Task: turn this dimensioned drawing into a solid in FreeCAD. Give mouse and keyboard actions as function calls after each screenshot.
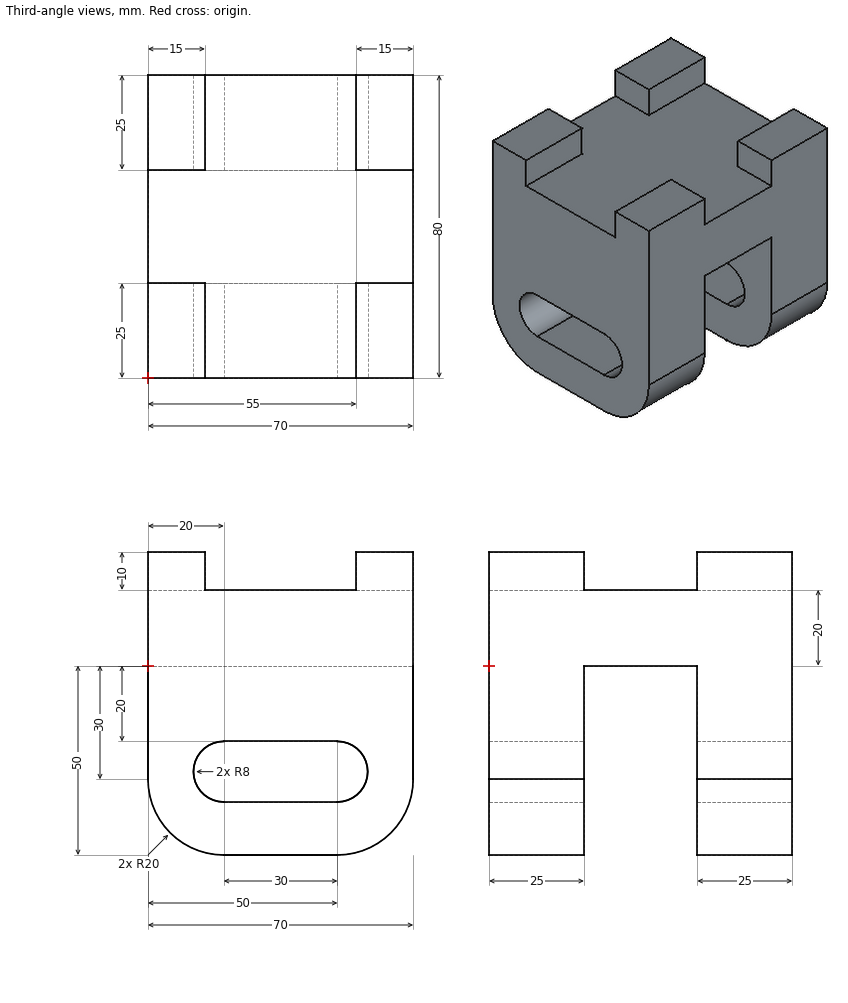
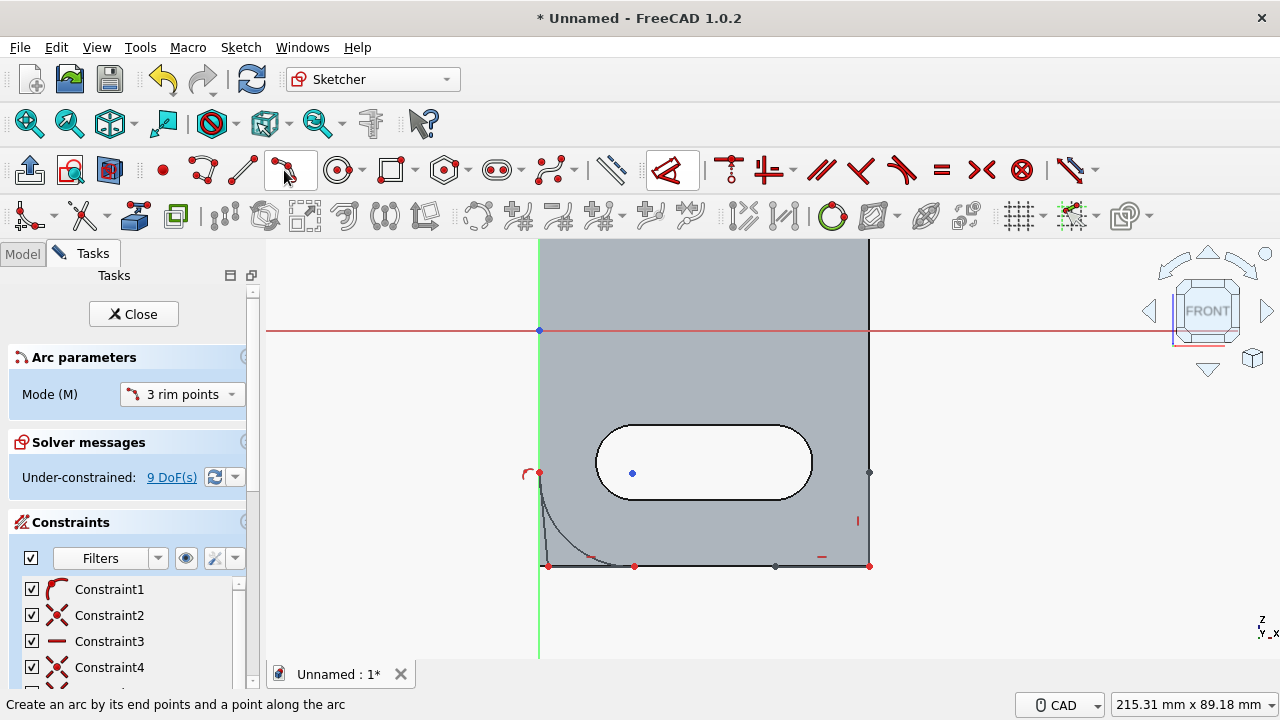
click(869, 473)
click(775, 567)
click(842, 539)
key(Escape)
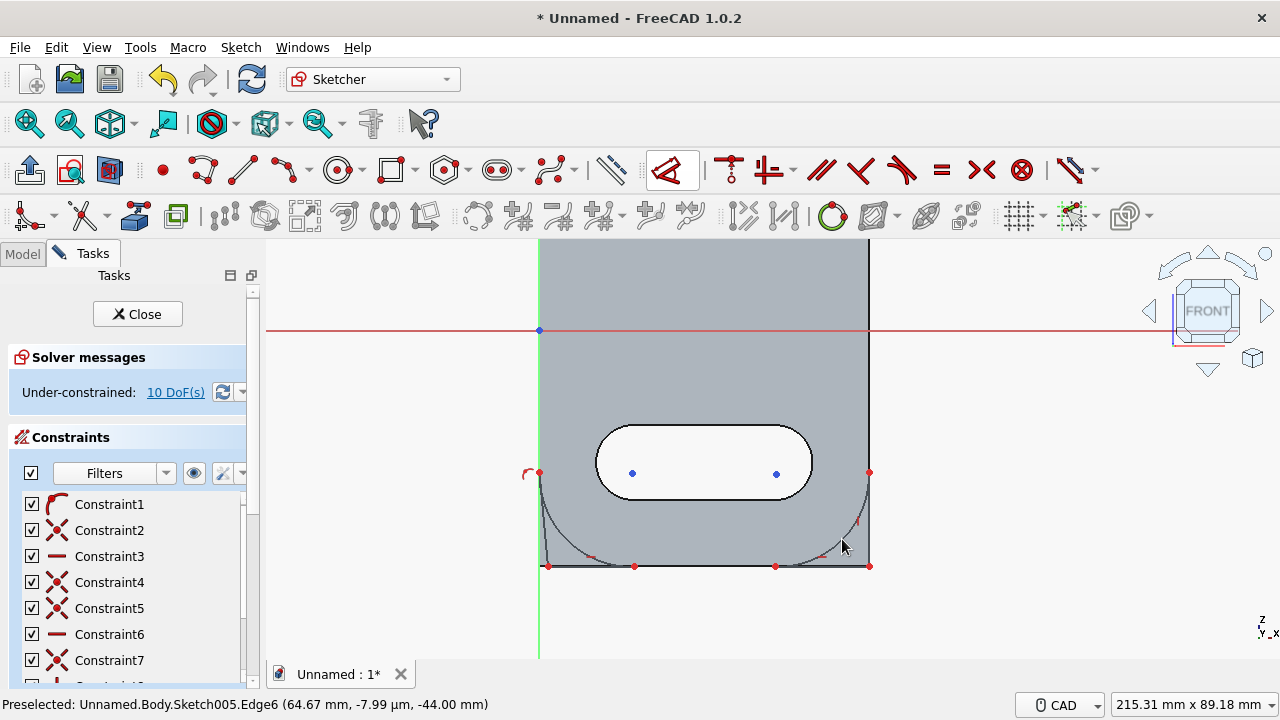
scroll(546, 548, up, 4)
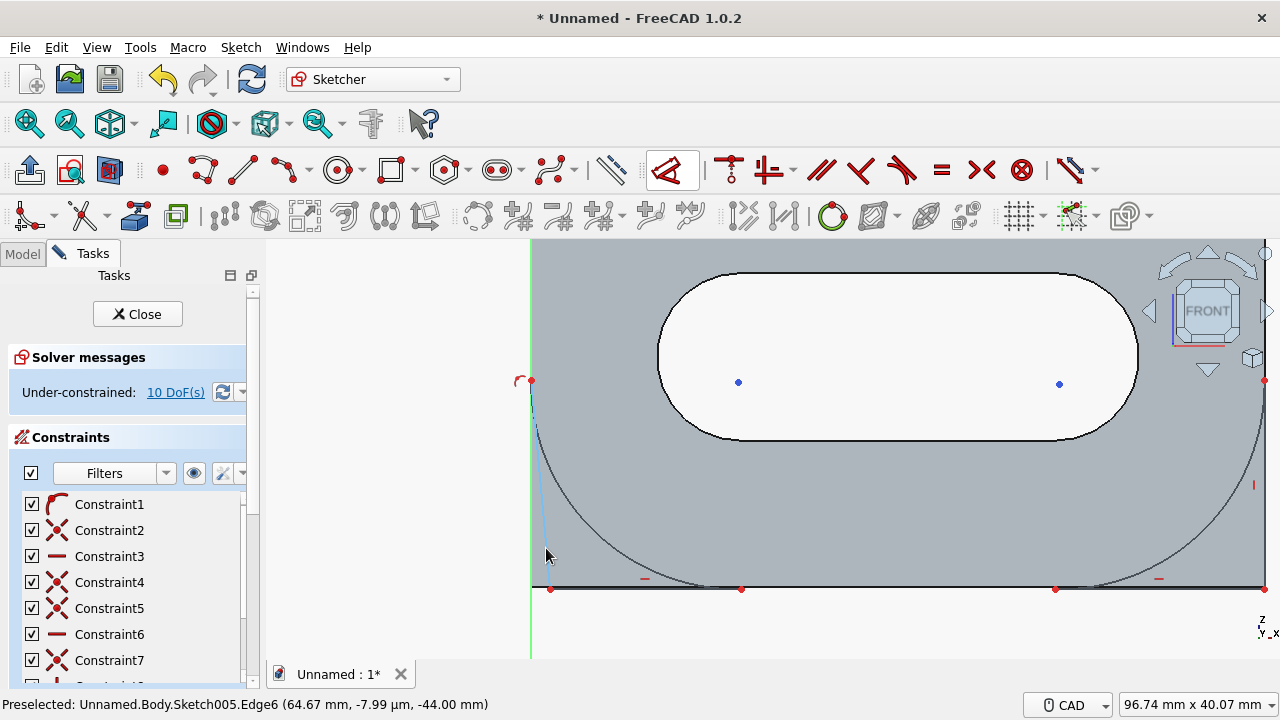
click(546, 548)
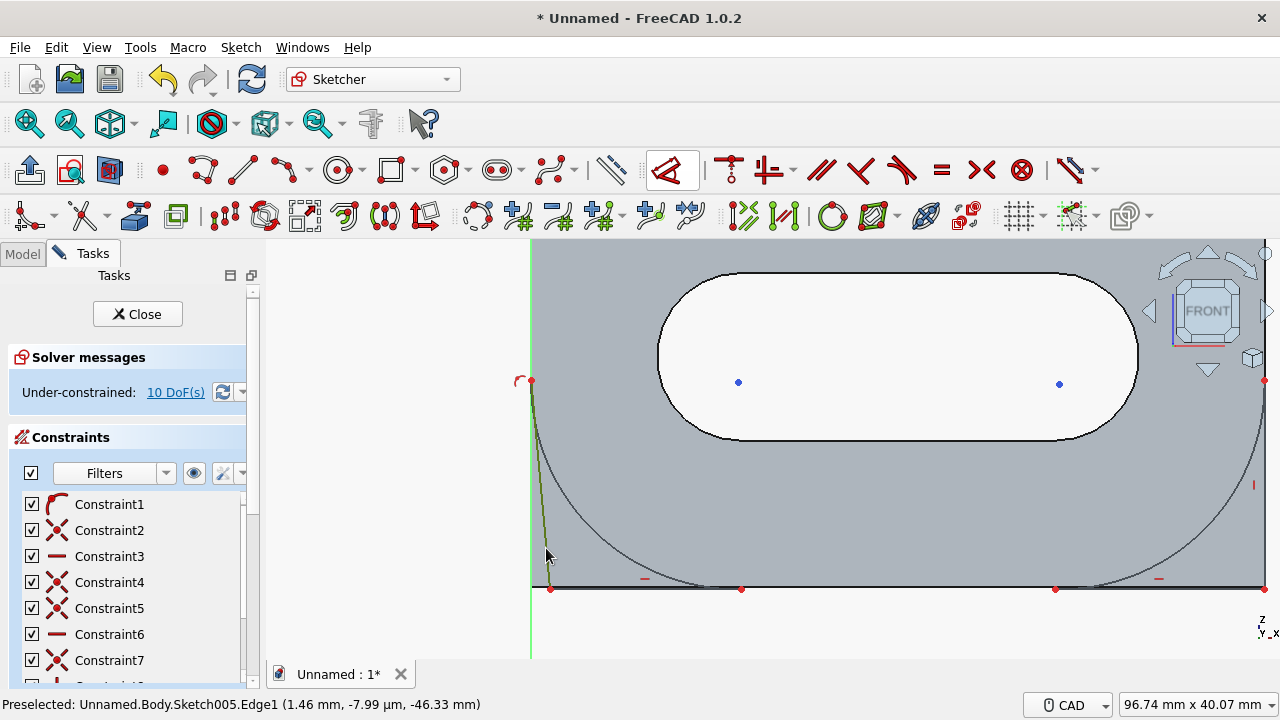
click(554, 476)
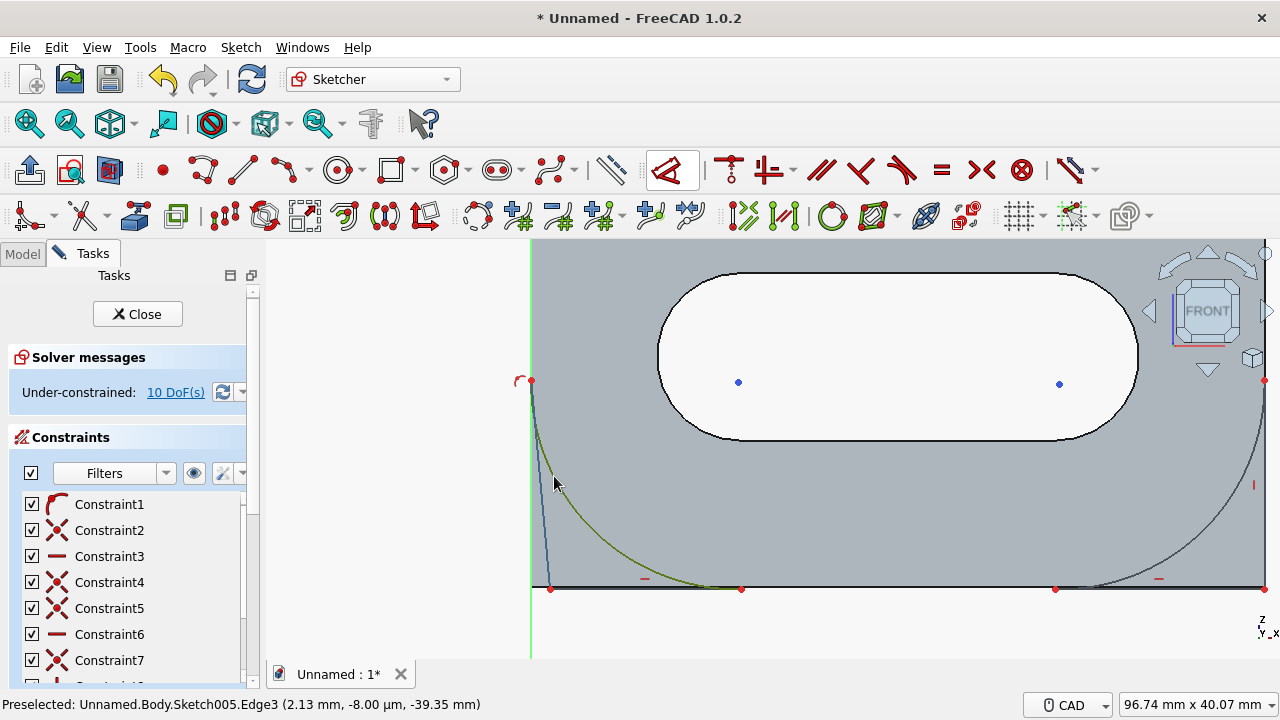
click(902, 170)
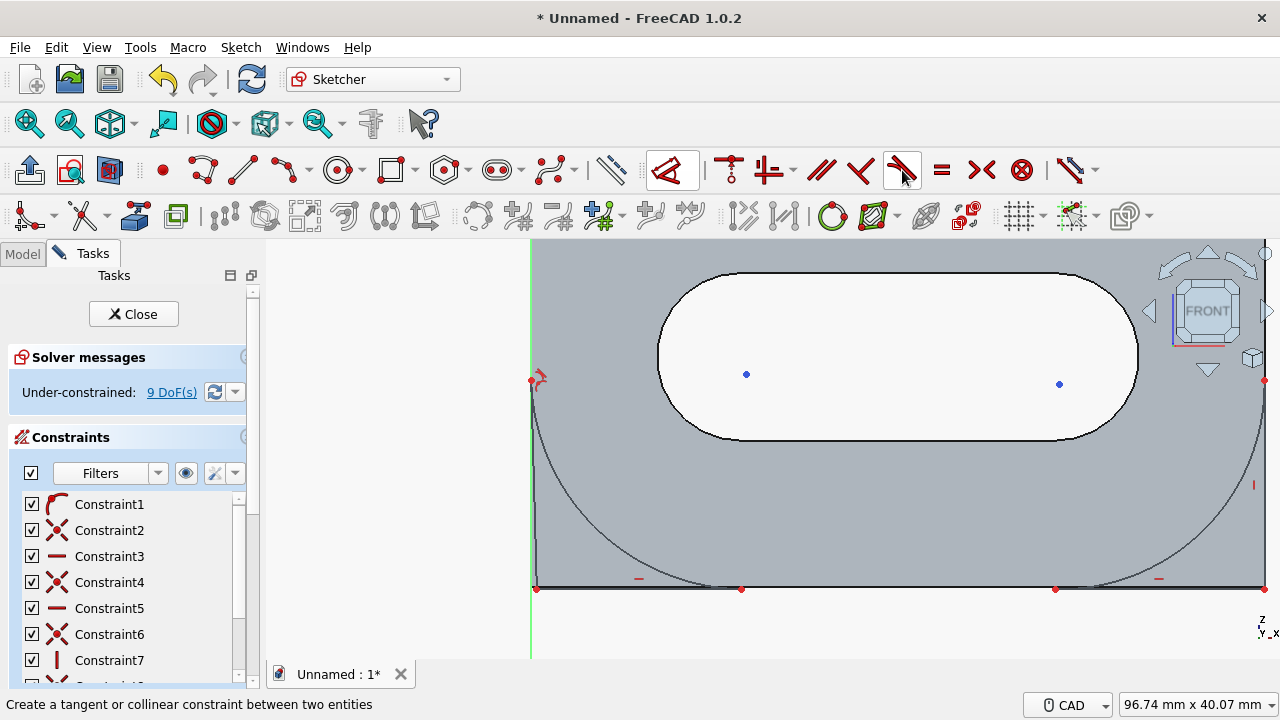
click(598, 589)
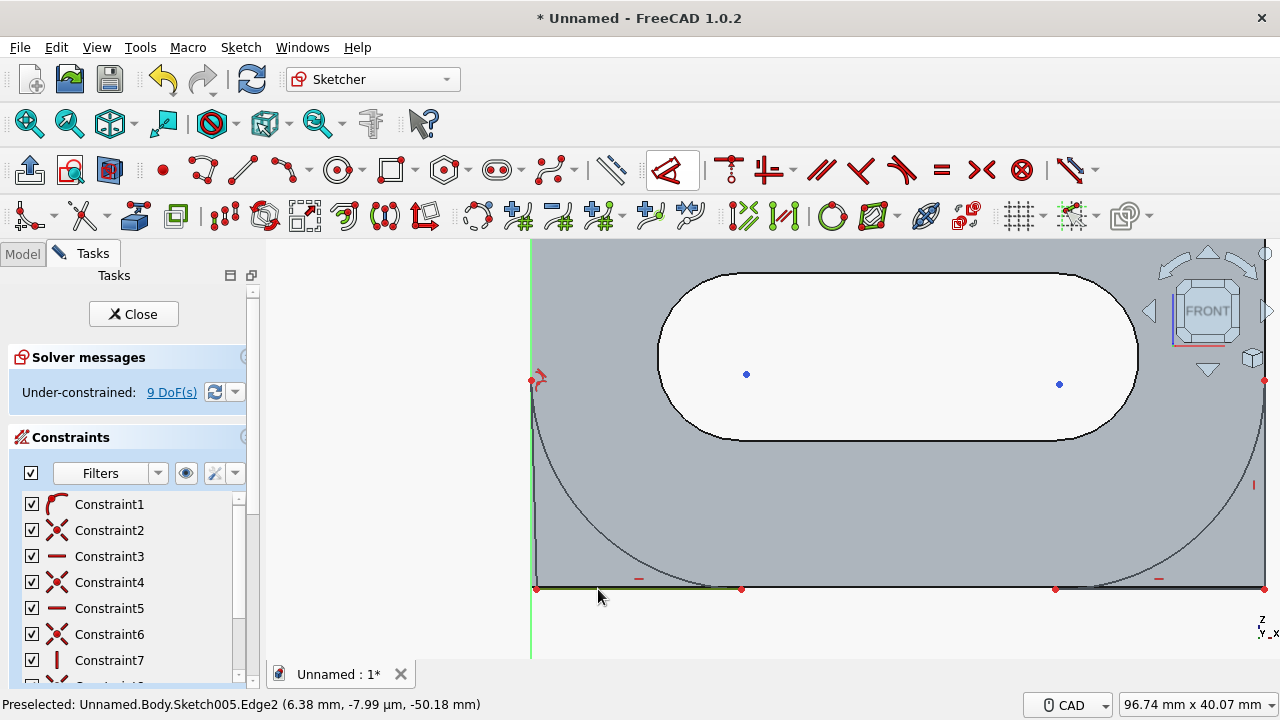
click(556, 474)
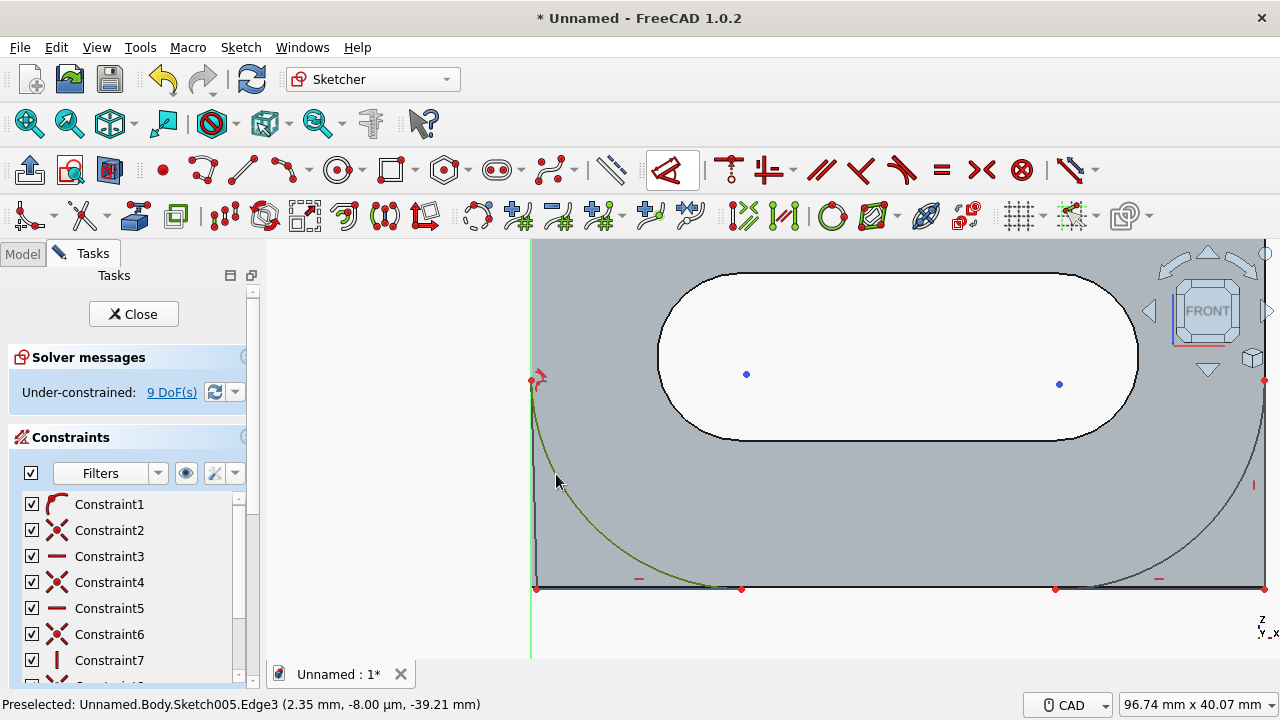
click(902, 170)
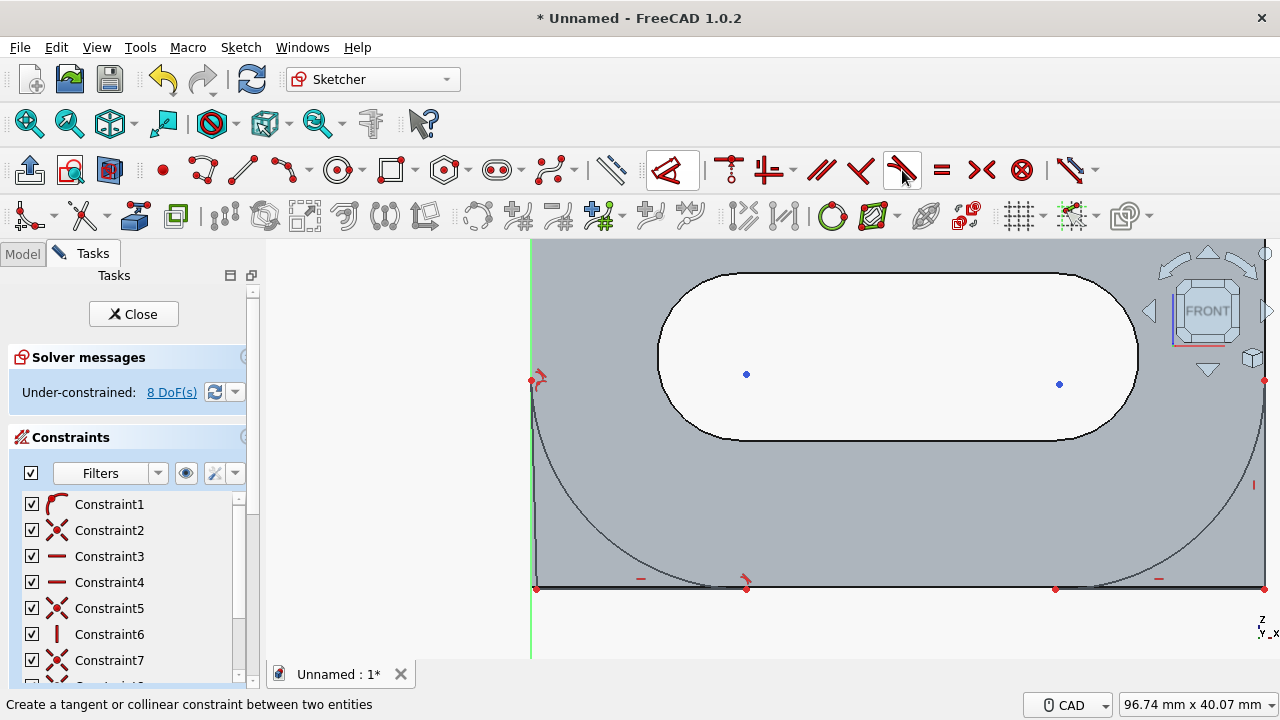
scroll(547, 550, down, 4)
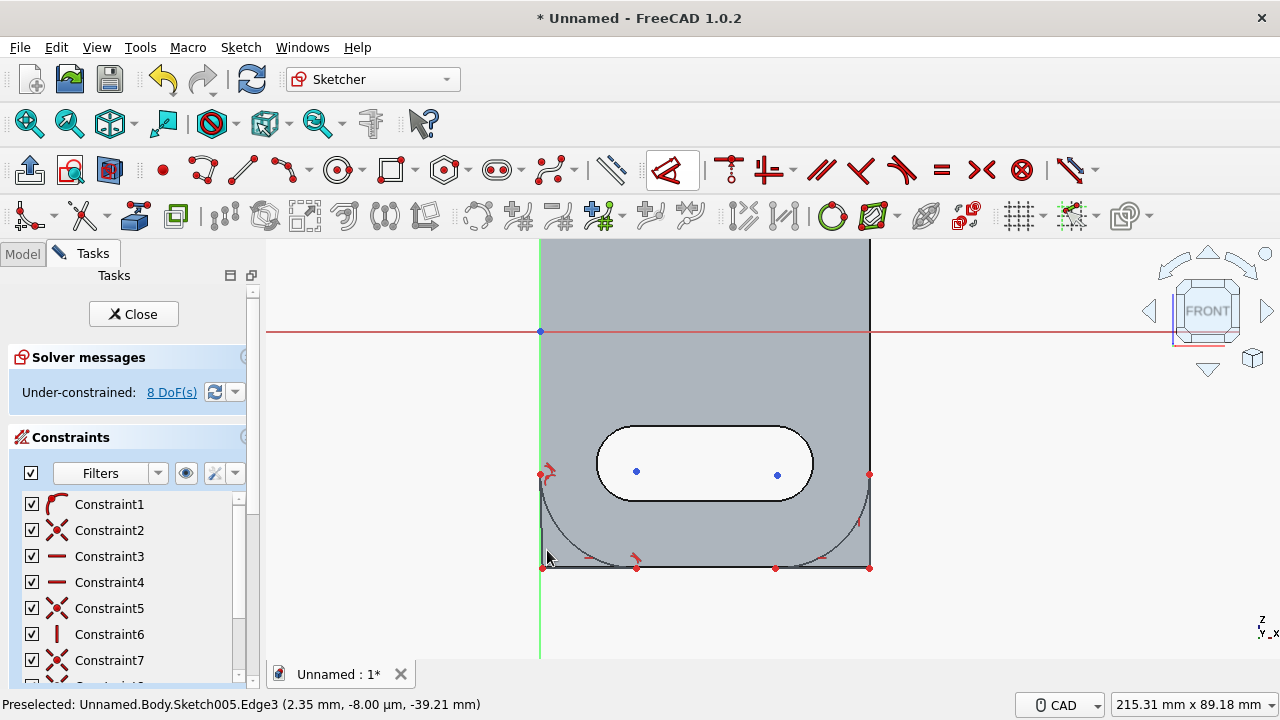
click(841, 568)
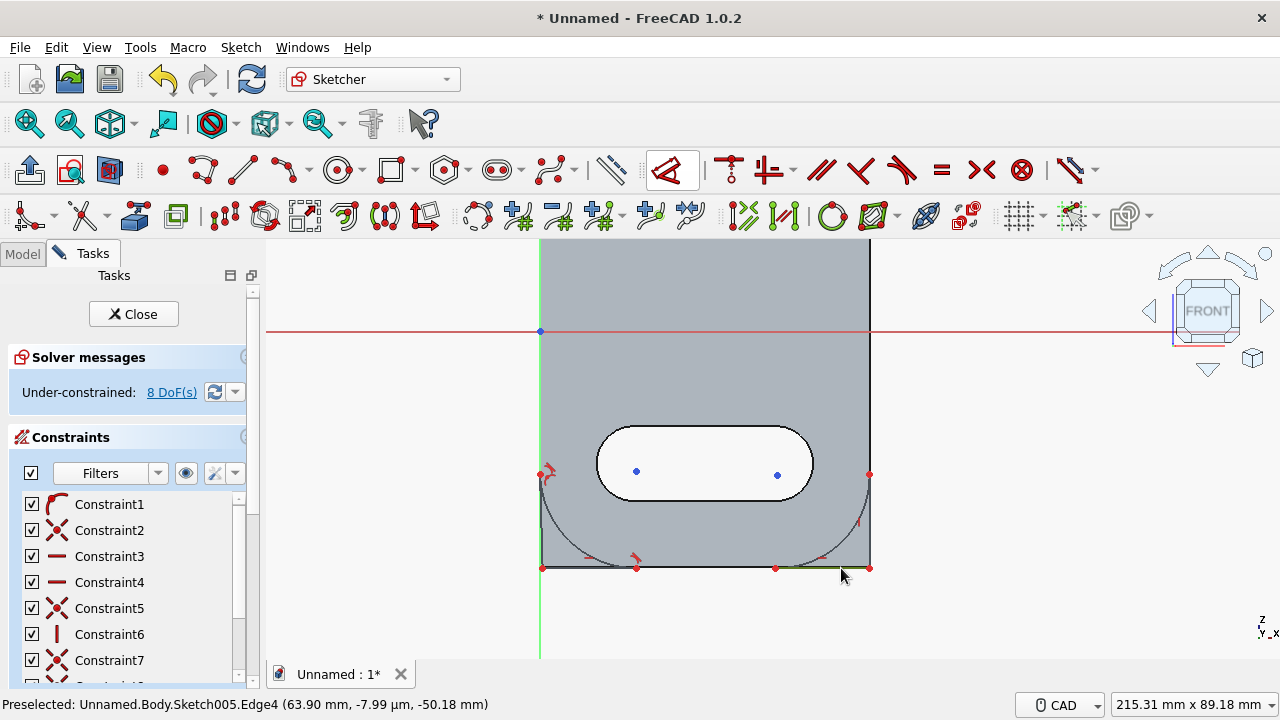
scroll(819, 558, up, 2)